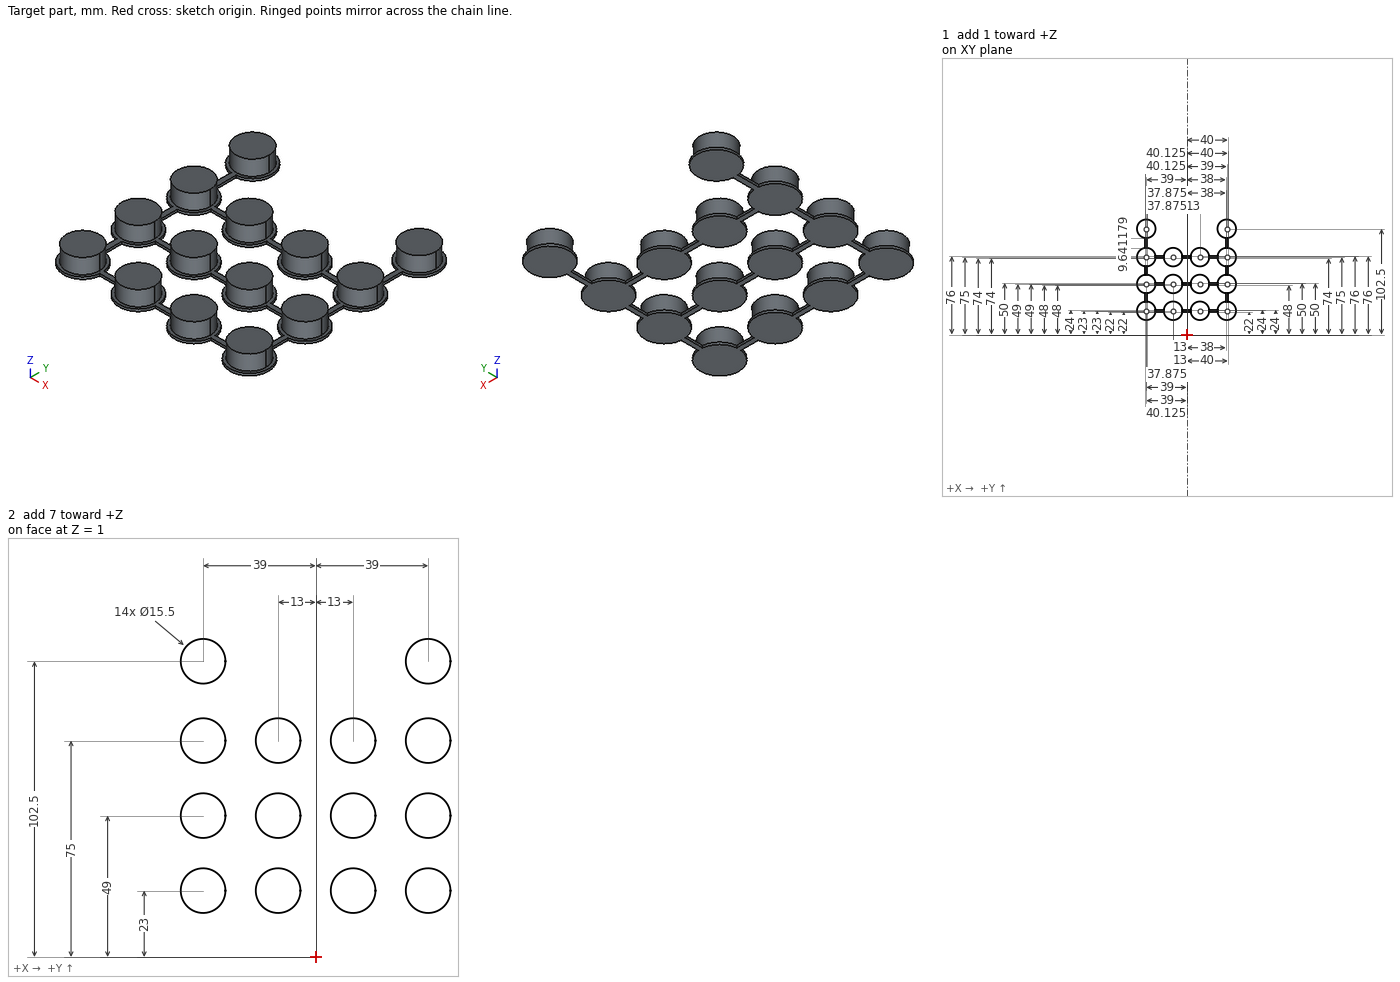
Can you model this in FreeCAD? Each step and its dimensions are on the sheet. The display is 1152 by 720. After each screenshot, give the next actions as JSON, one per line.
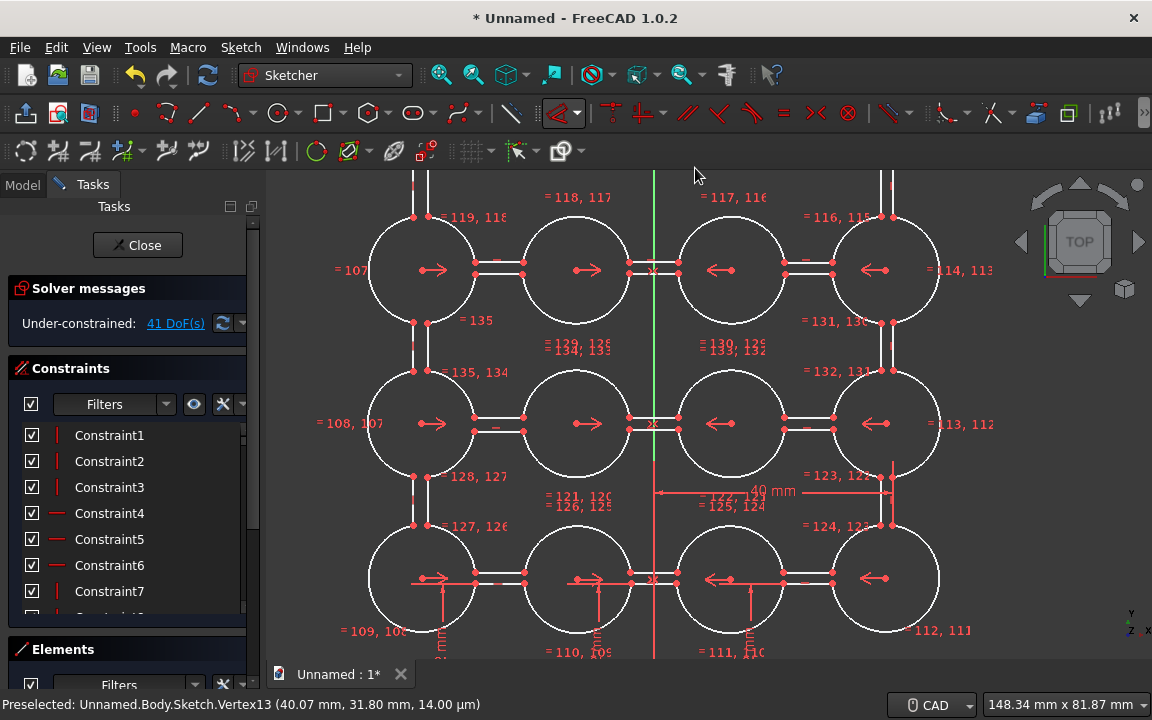
{"action": "left_click", "coordinate": [893, 371]}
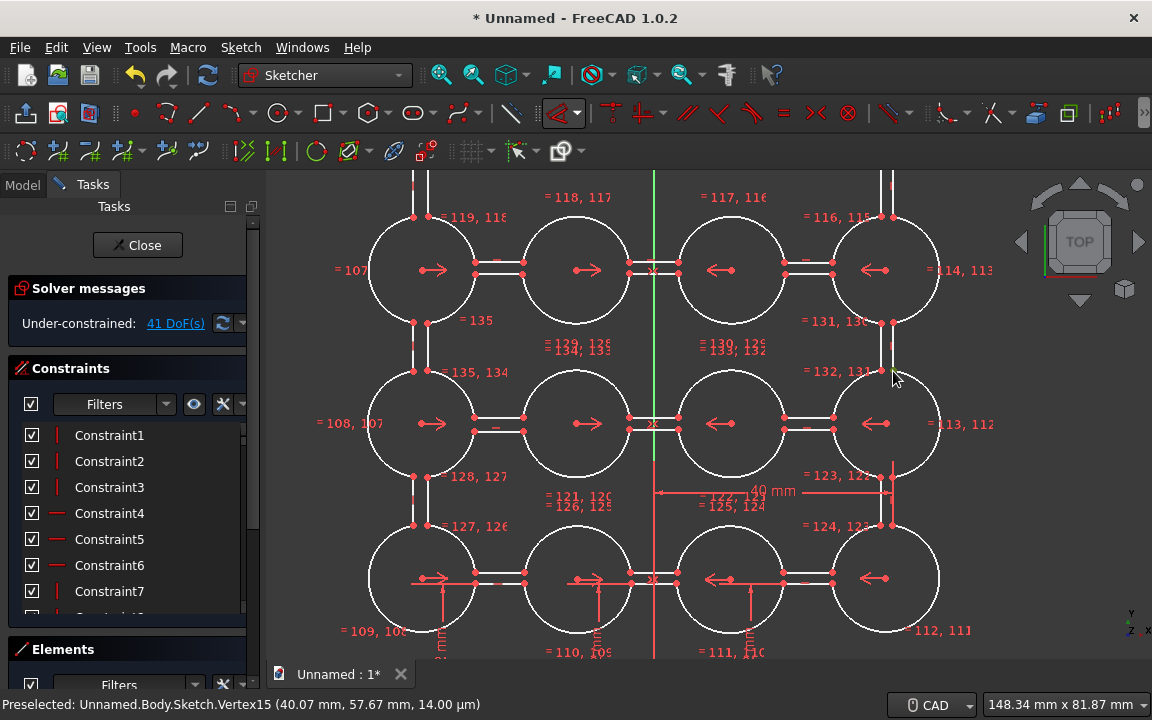
{"action": "left_click", "coordinate": [580, 114]}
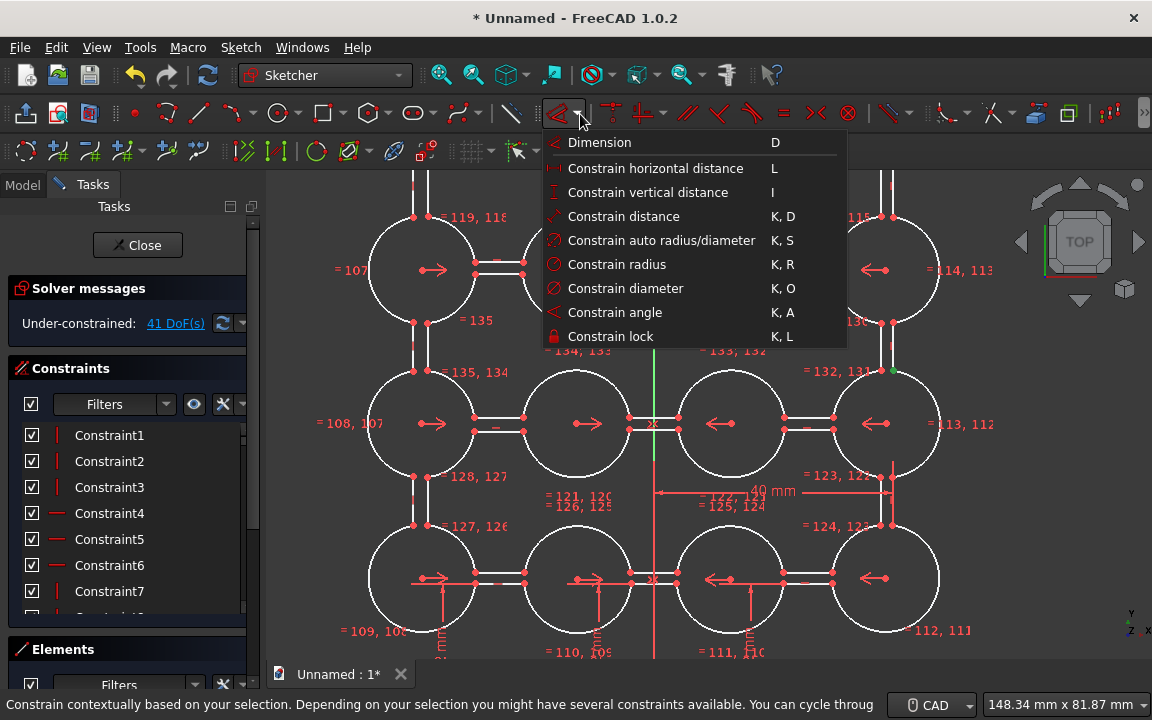
{"action": "left_click", "coordinate": [695, 168]}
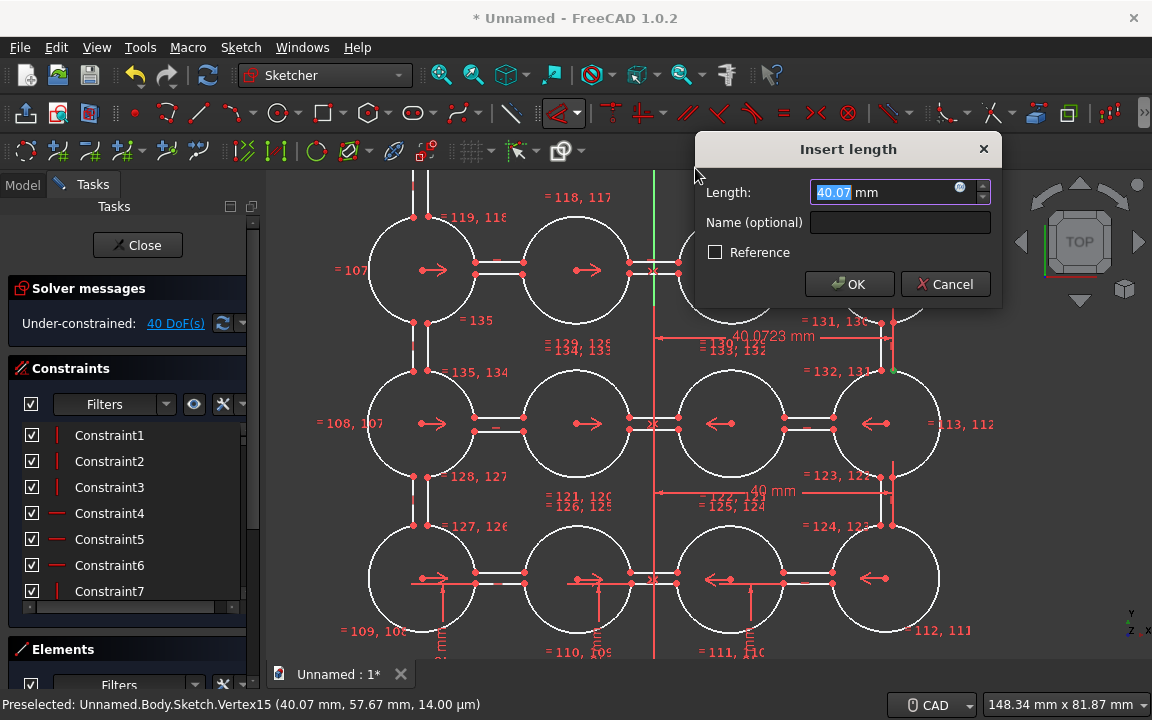
{"action": "type", "text": "40"}
{"action": "key", "text": "Return"}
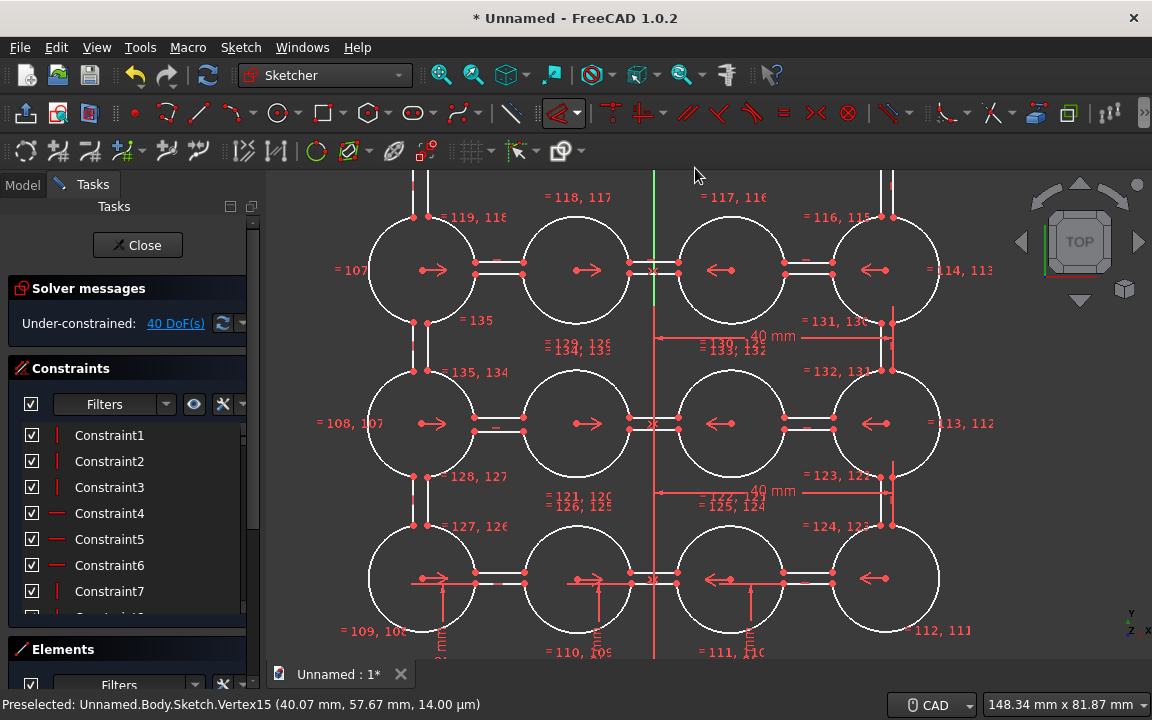
{"action": "left_click", "coordinate": [893, 217]}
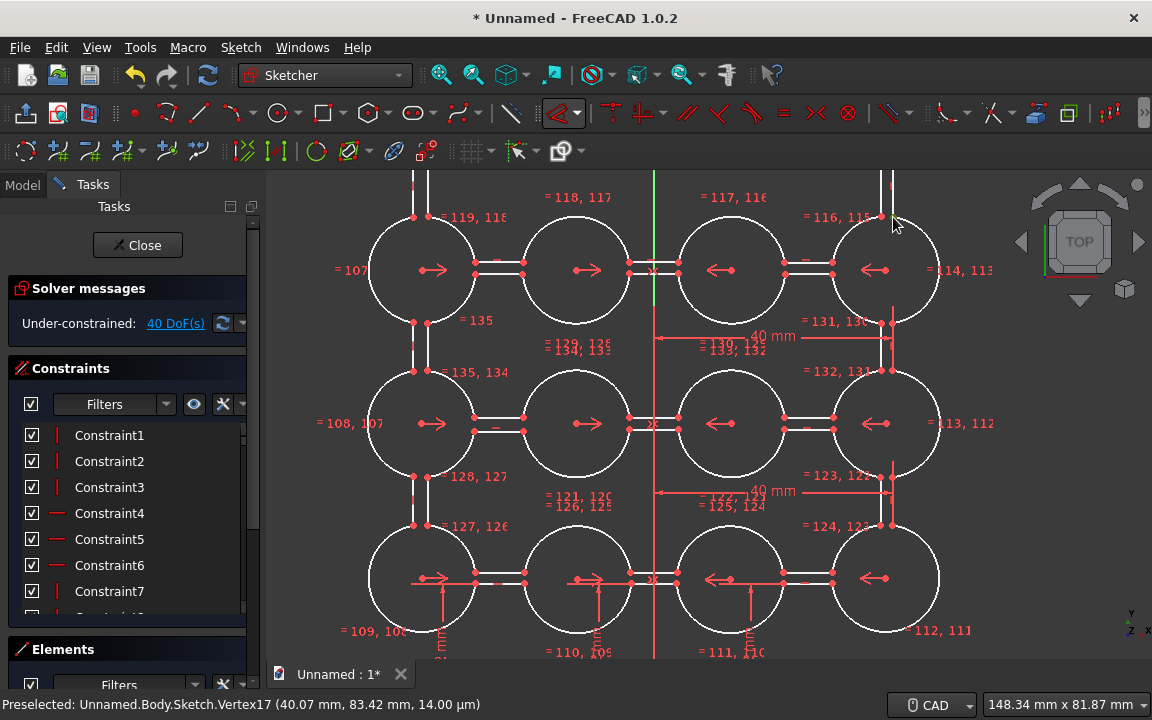
{"action": "left_click", "coordinate": [580, 114]}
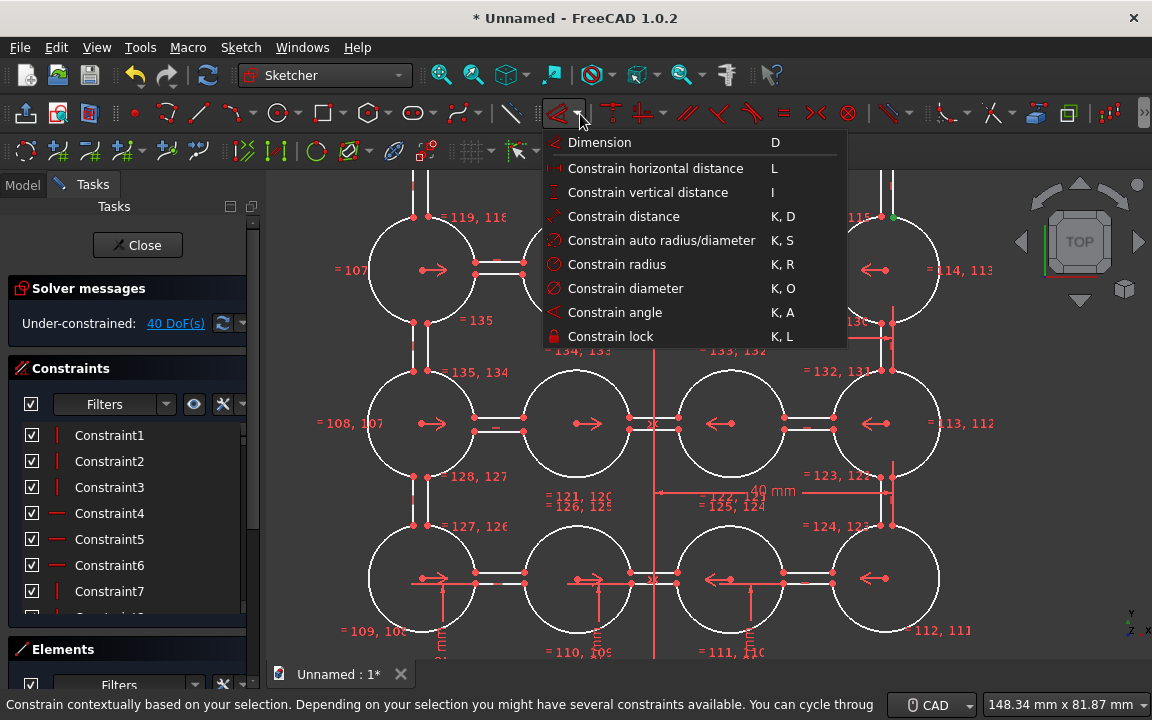
{"action": "left_click", "coordinate": [695, 168]}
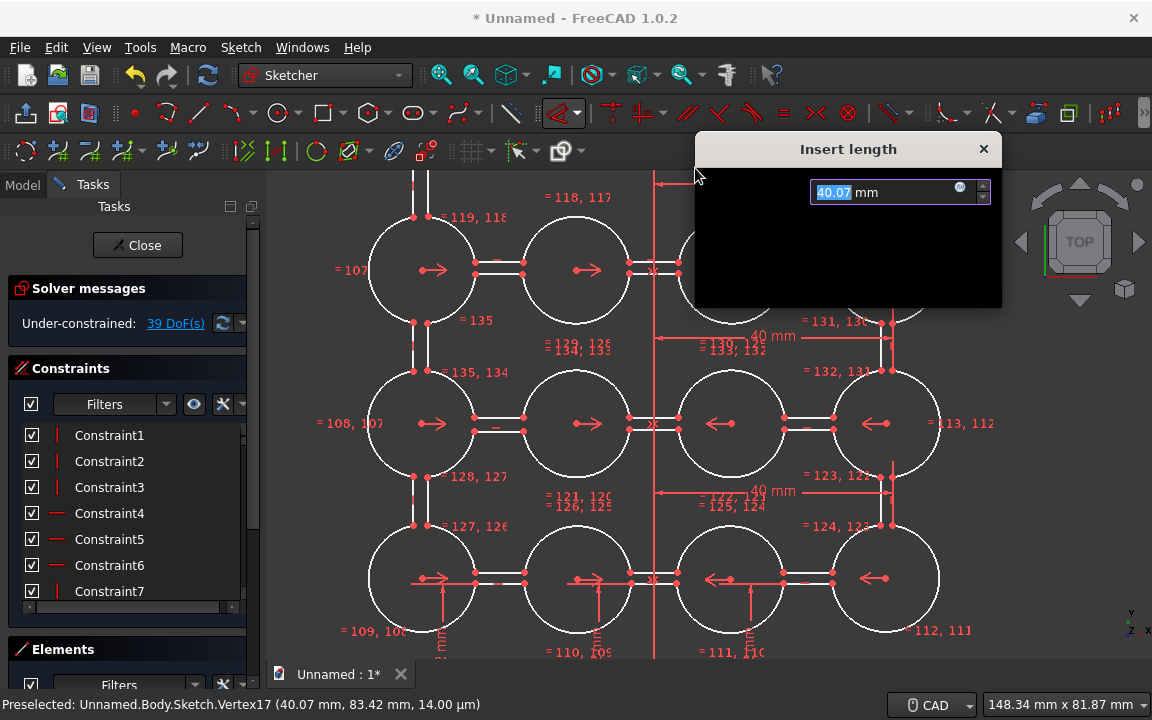
{"action": "type", "text": "40"}
{"action": "key", "text": "Return"}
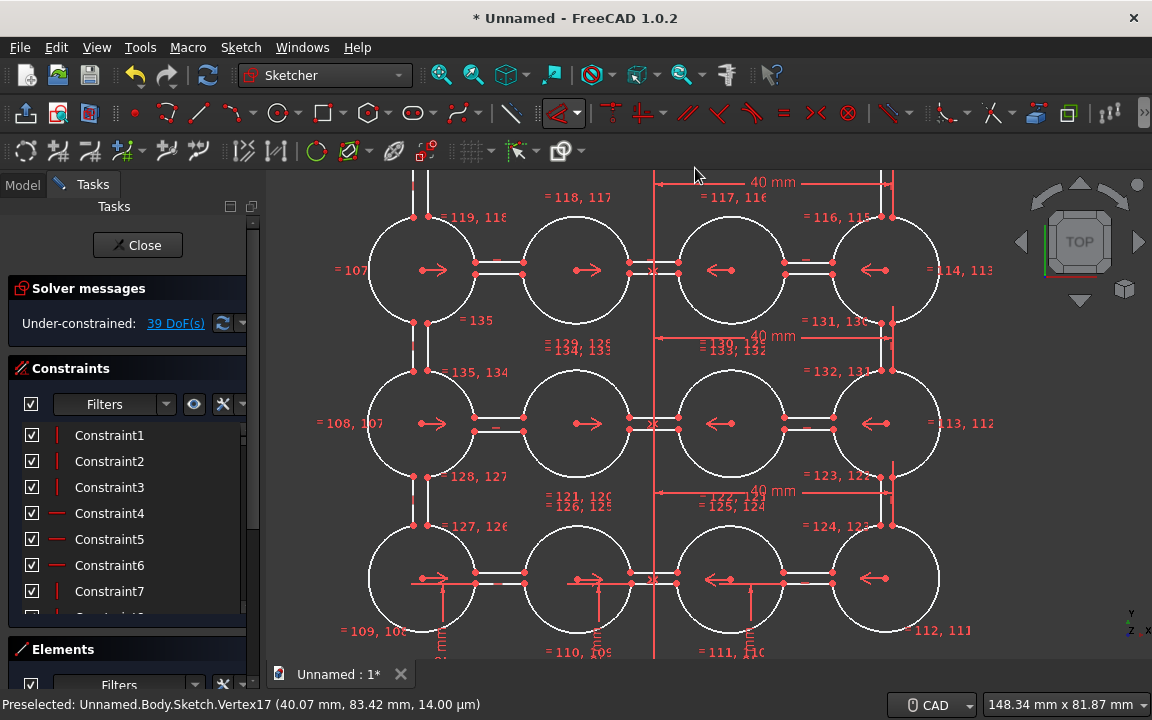
{"action": "scroll", "coordinate": [630, 441], "scroll_direction": "down", "scroll_amount": 4}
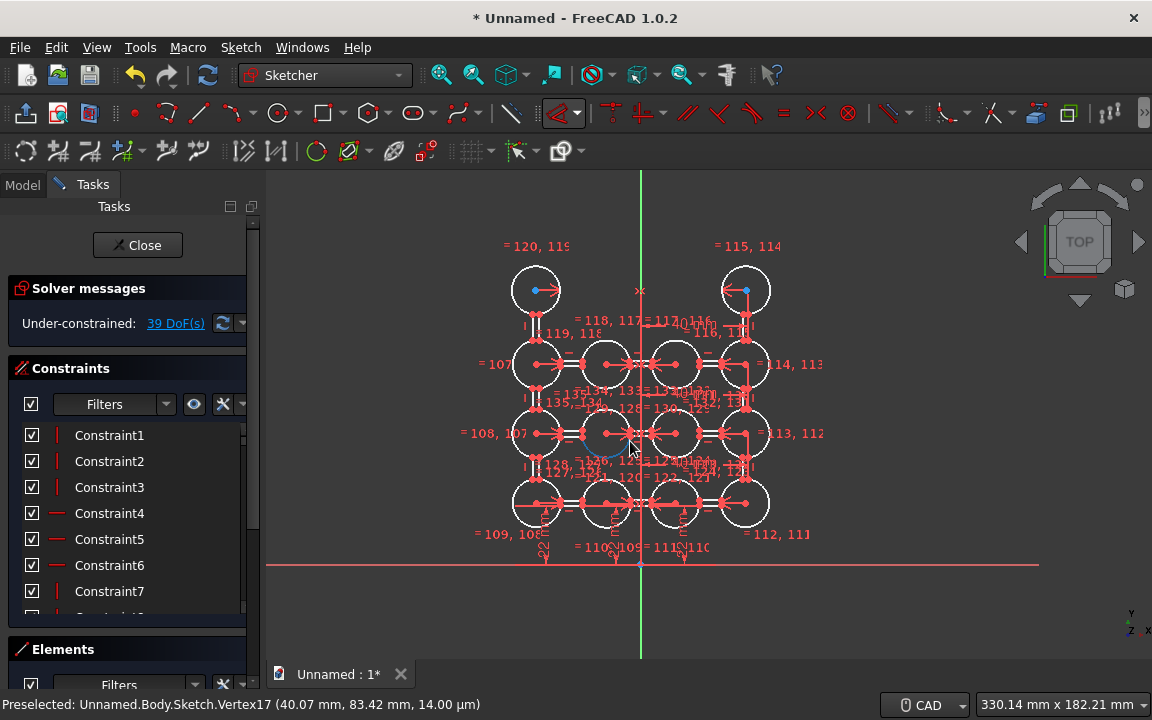
{"action": "scroll", "coordinate": [743, 314], "scroll_direction": "up", "scroll_amount": 5}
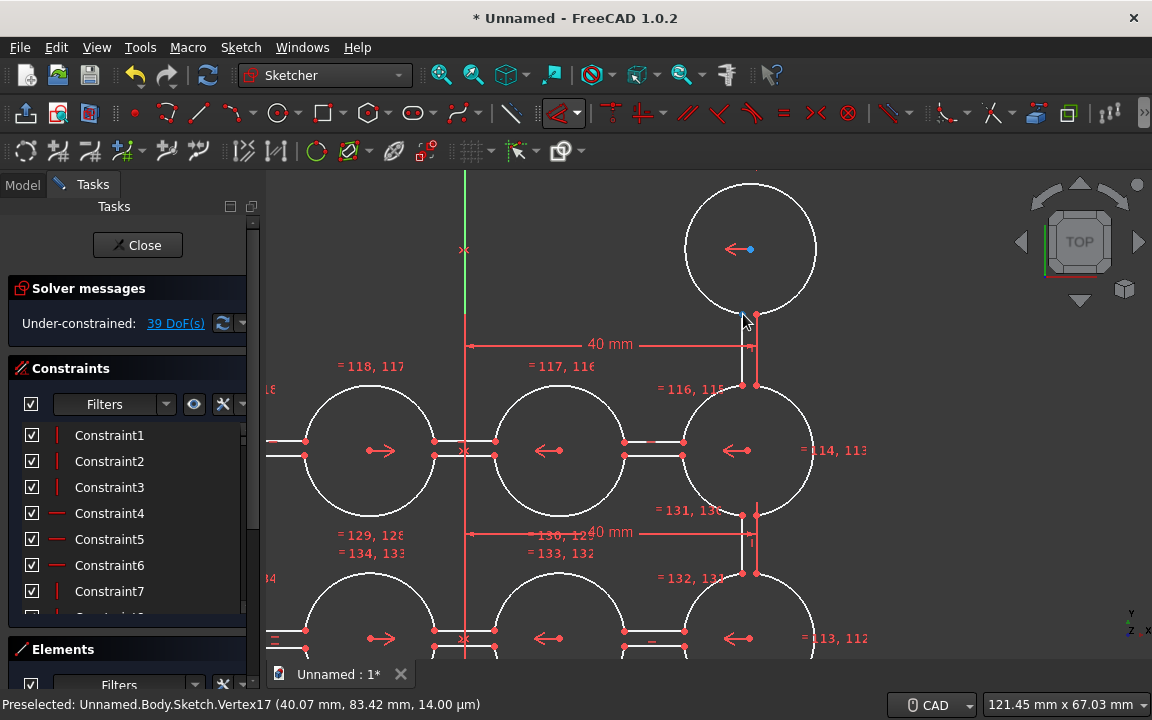
{"action": "left_click", "coordinate": [742, 314]}